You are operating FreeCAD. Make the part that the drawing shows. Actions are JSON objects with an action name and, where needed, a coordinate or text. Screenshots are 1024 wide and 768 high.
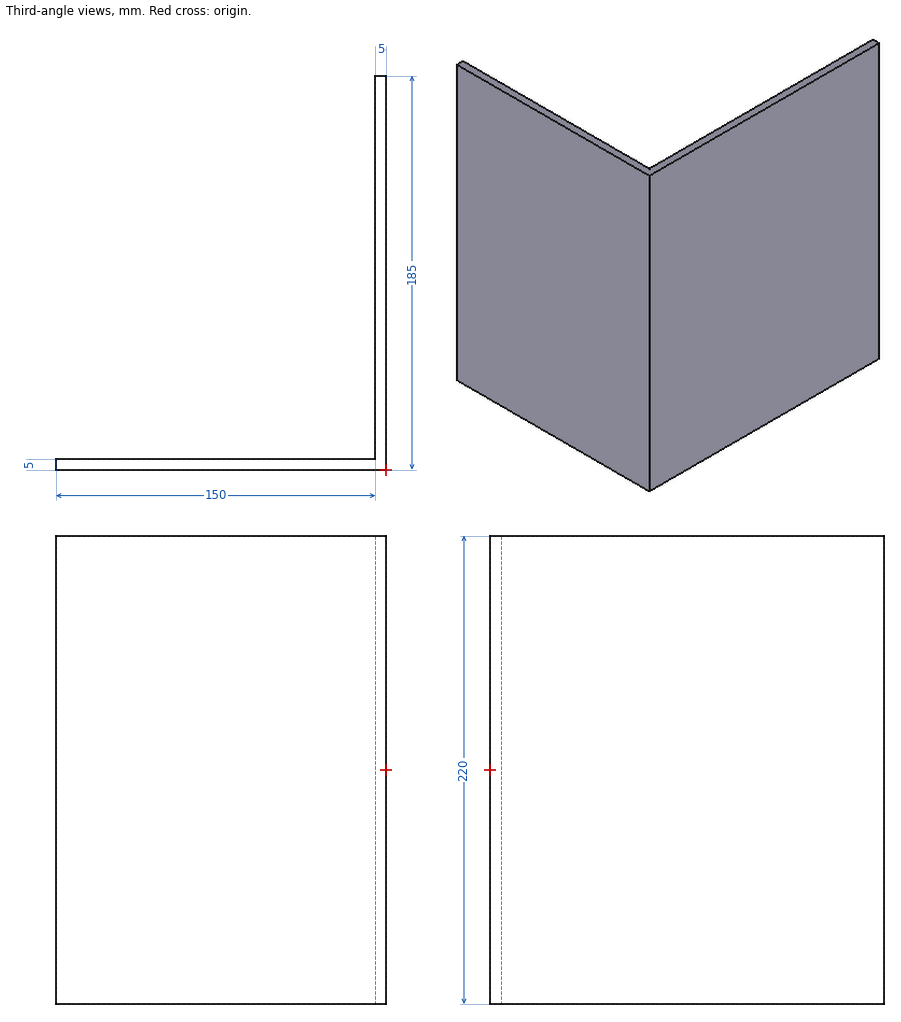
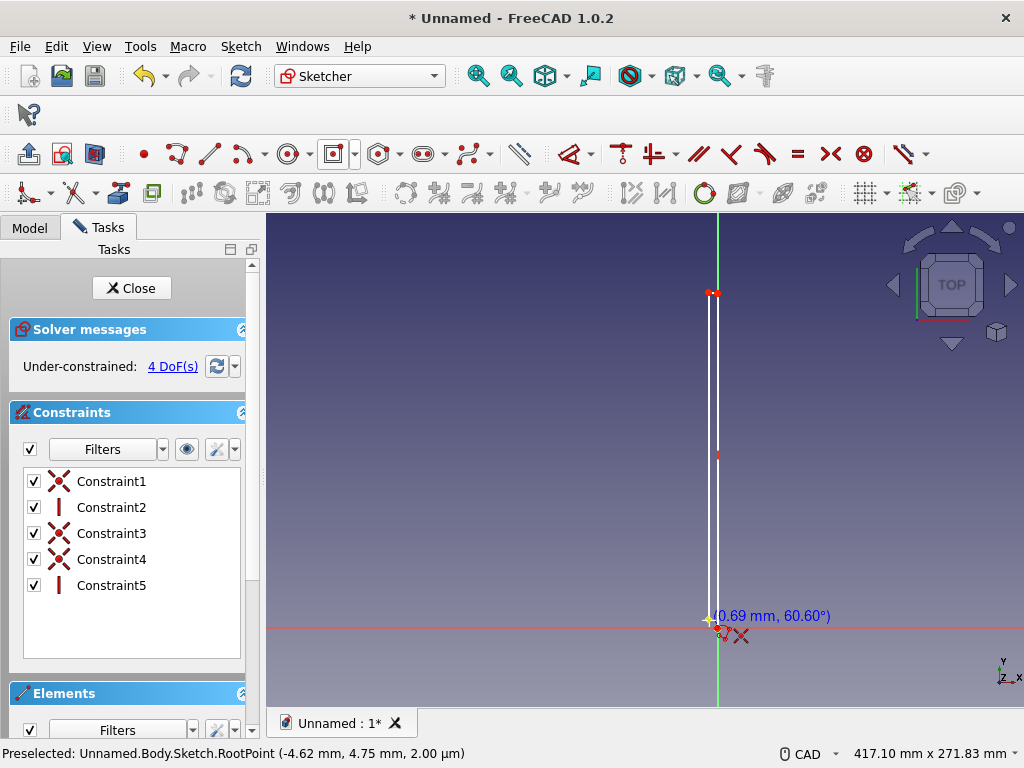
{"action": "scroll", "coordinate": [436, 619], "scroll_direction": "up", "scroll_amount": 3}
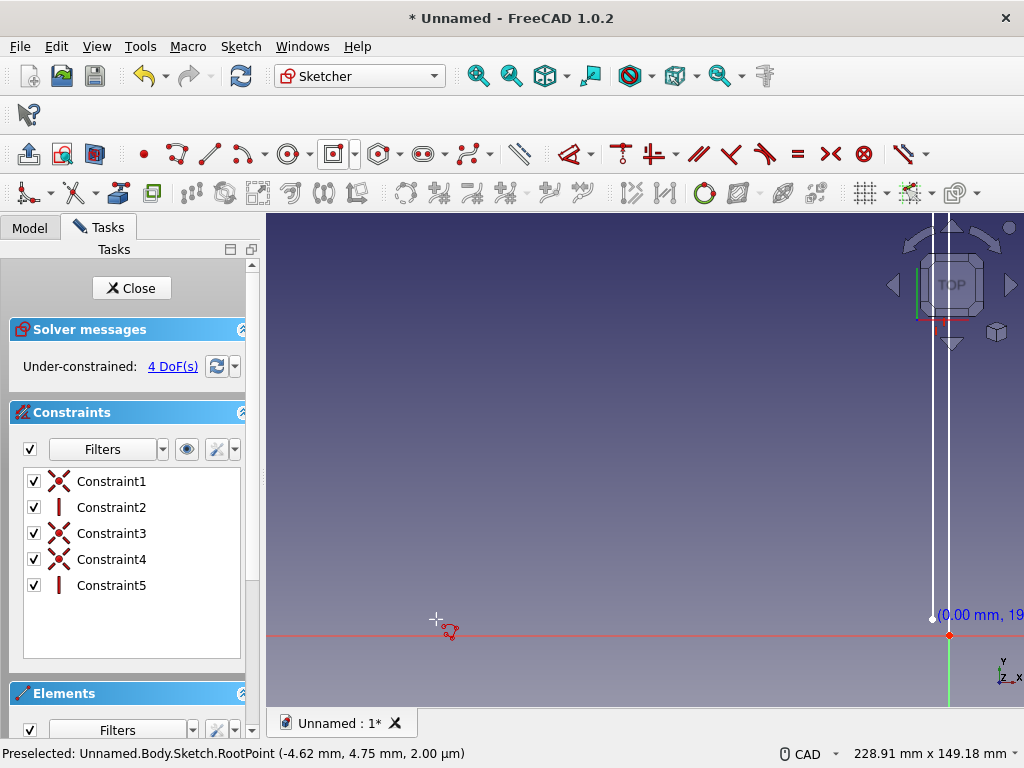
{"action": "left_click", "coordinate": [436, 619]}
{"action": "left_click", "coordinate": [436, 627]}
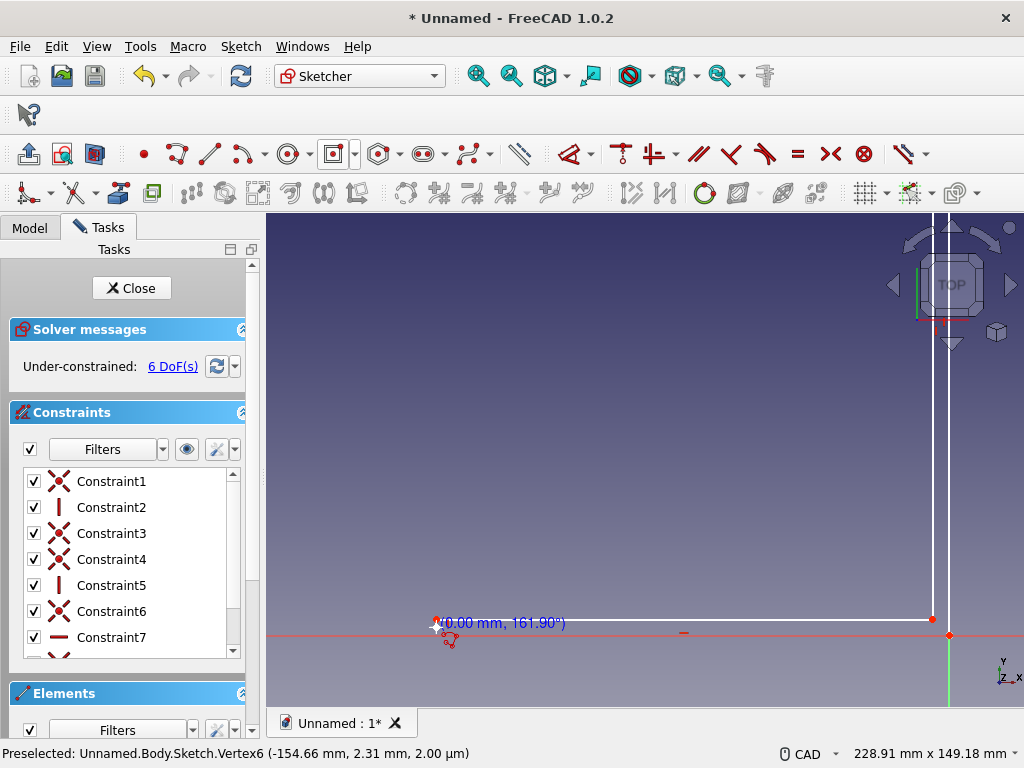
{"action": "scroll", "coordinate": [436, 619], "scroll_direction": "down", "scroll_amount": 3}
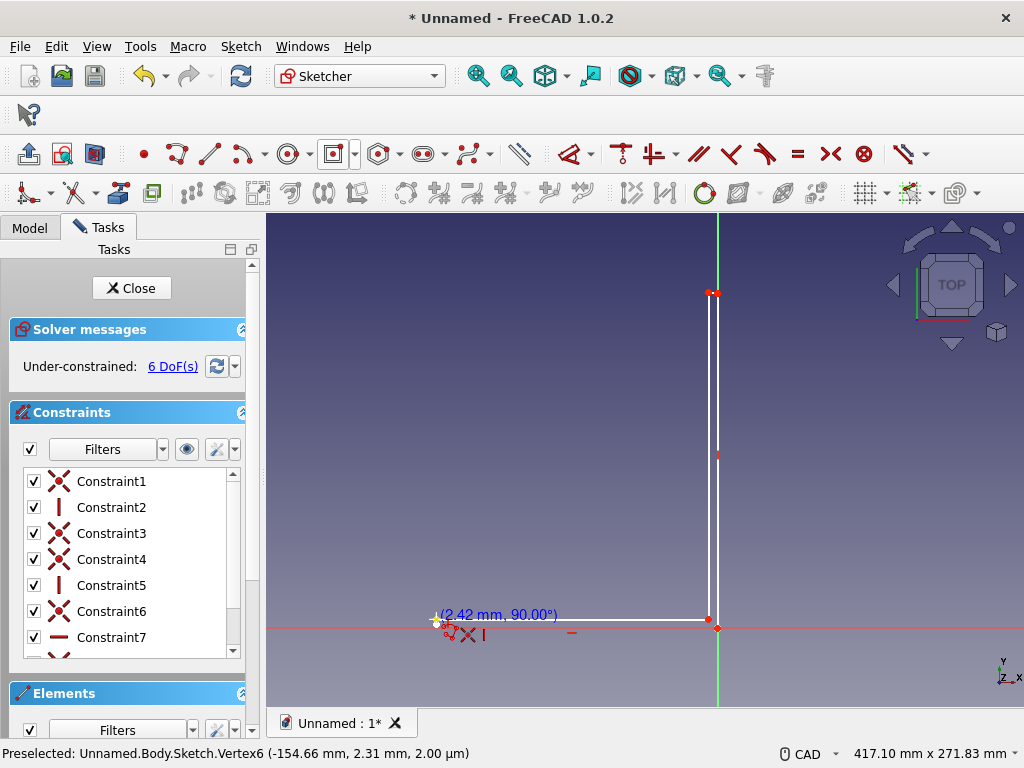
{"action": "scroll", "coordinate": [718, 628], "scroll_direction": "up", "scroll_amount": 2}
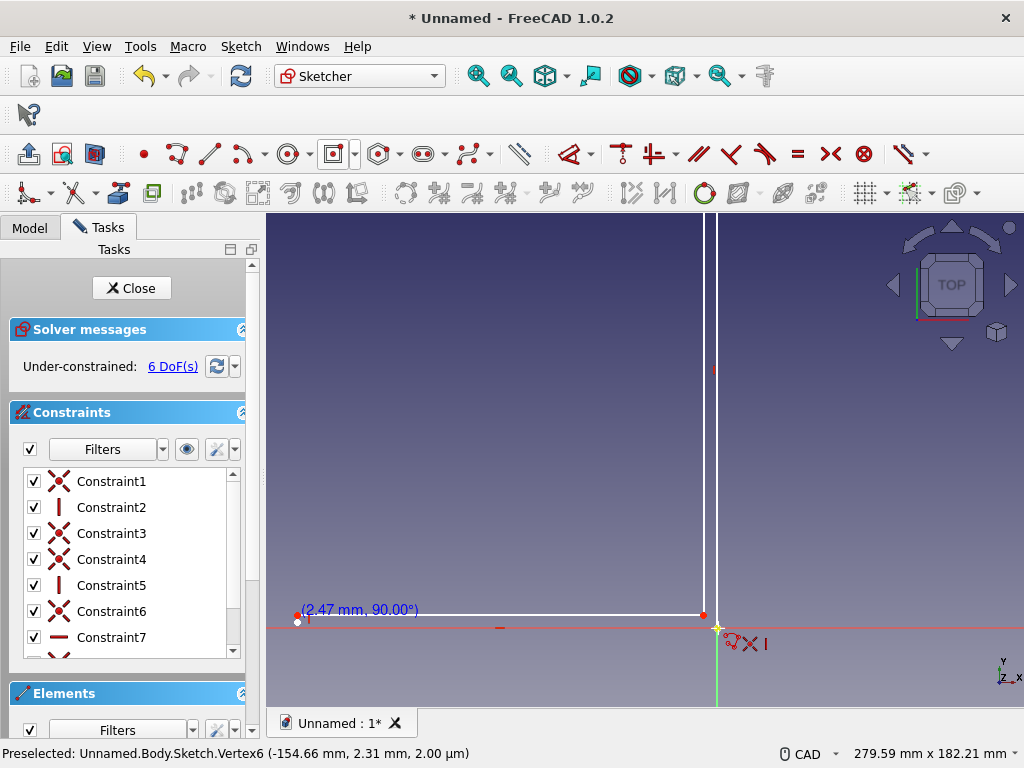
{"action": "left_click", "coordinate": [717, 628]}
{"action": "key", "text": "Escape"}
{"action": "key", "text": "Escape"}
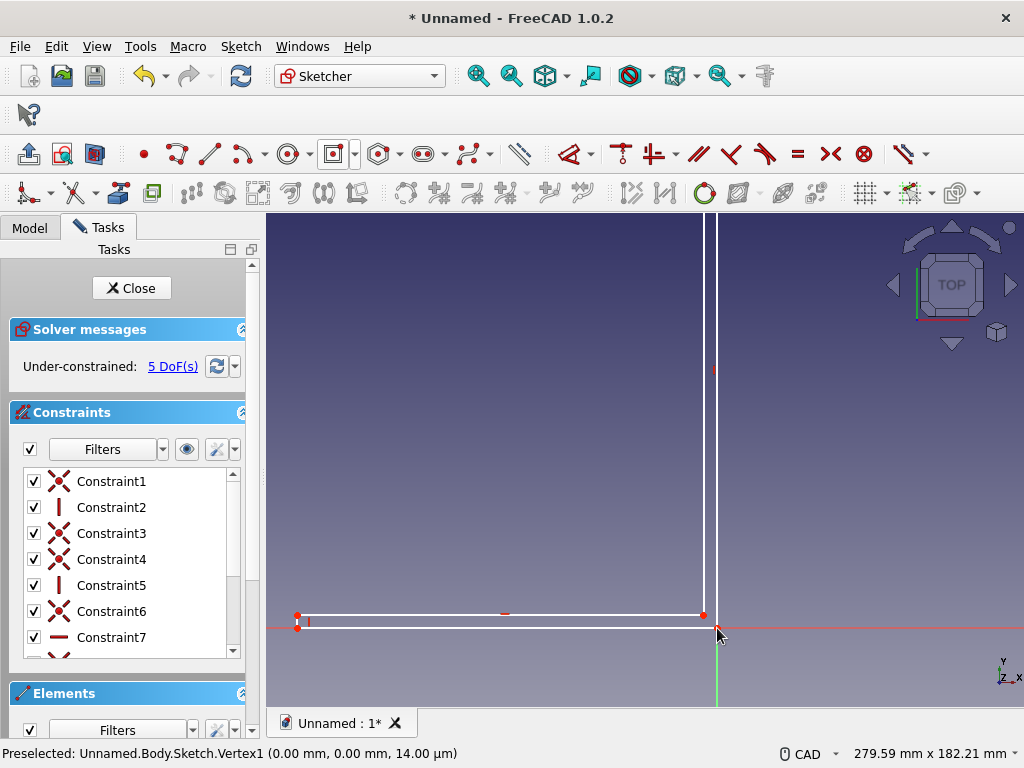
{"action": "scroll", "coordinate": [718, 628], "scroll_direction": "down", "scroll_amount": 2}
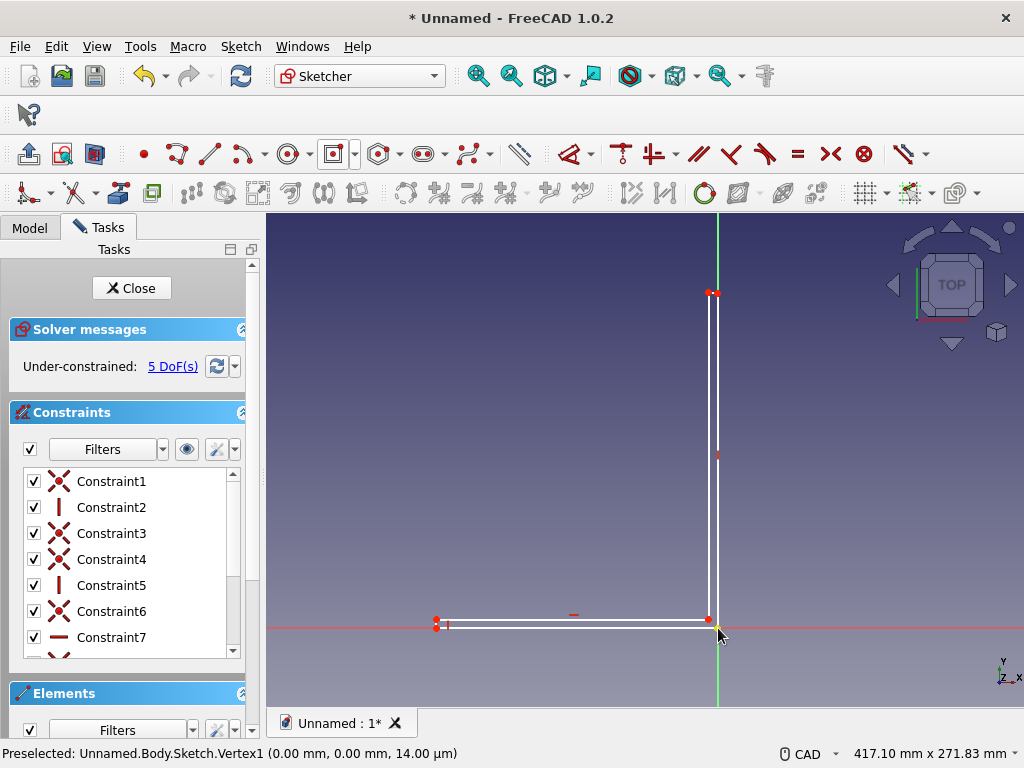
{"action": "scroll", "coordinate": [713, 293], "scroll_direction": "up", "scroll_amount": 6}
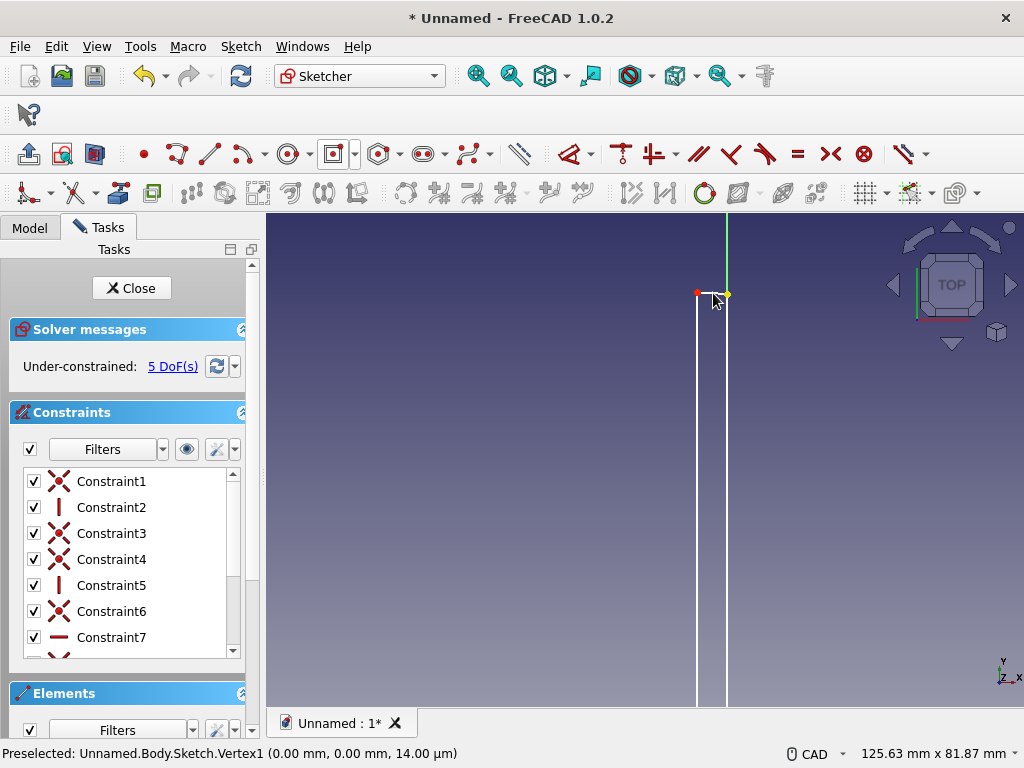
{"action": "left_click", "coordinate": [712, 293]}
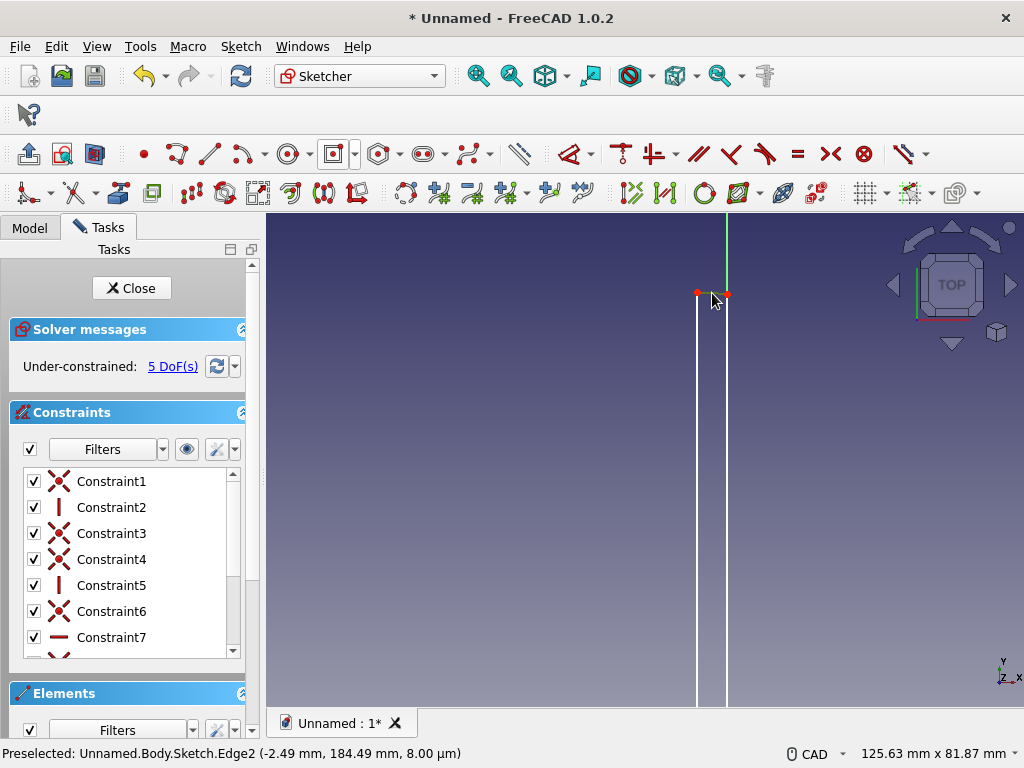
{"action": "left_click", "coordinate": [676, 154]}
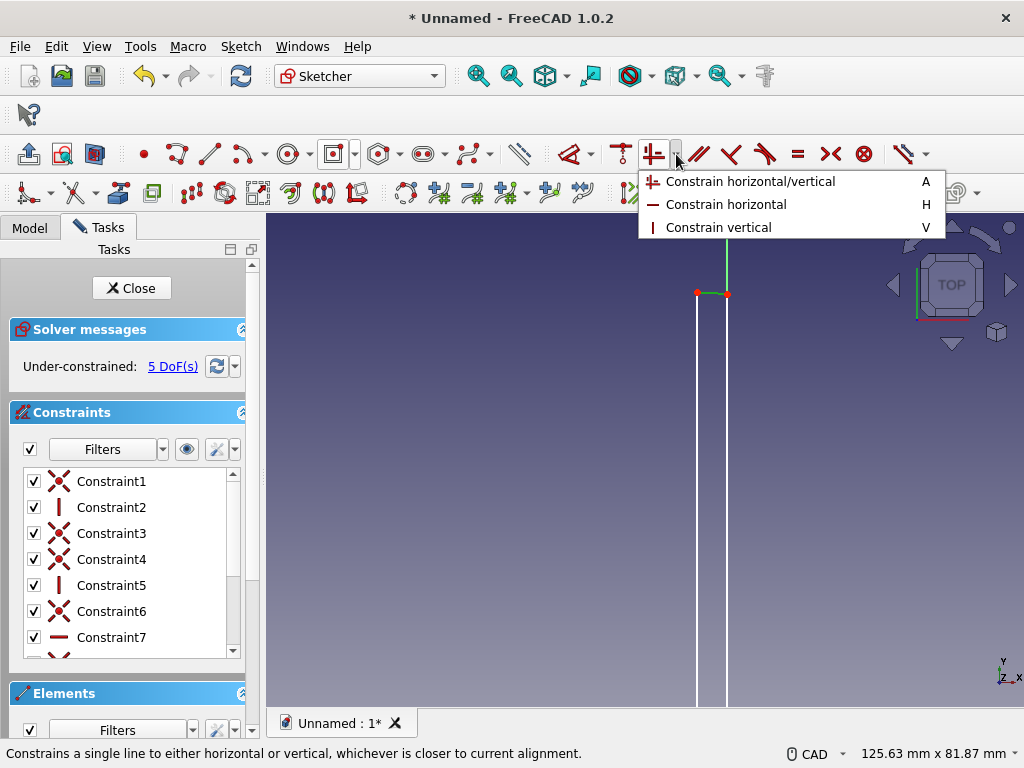
{"action": "left_click", "coordinate": [792, 204]}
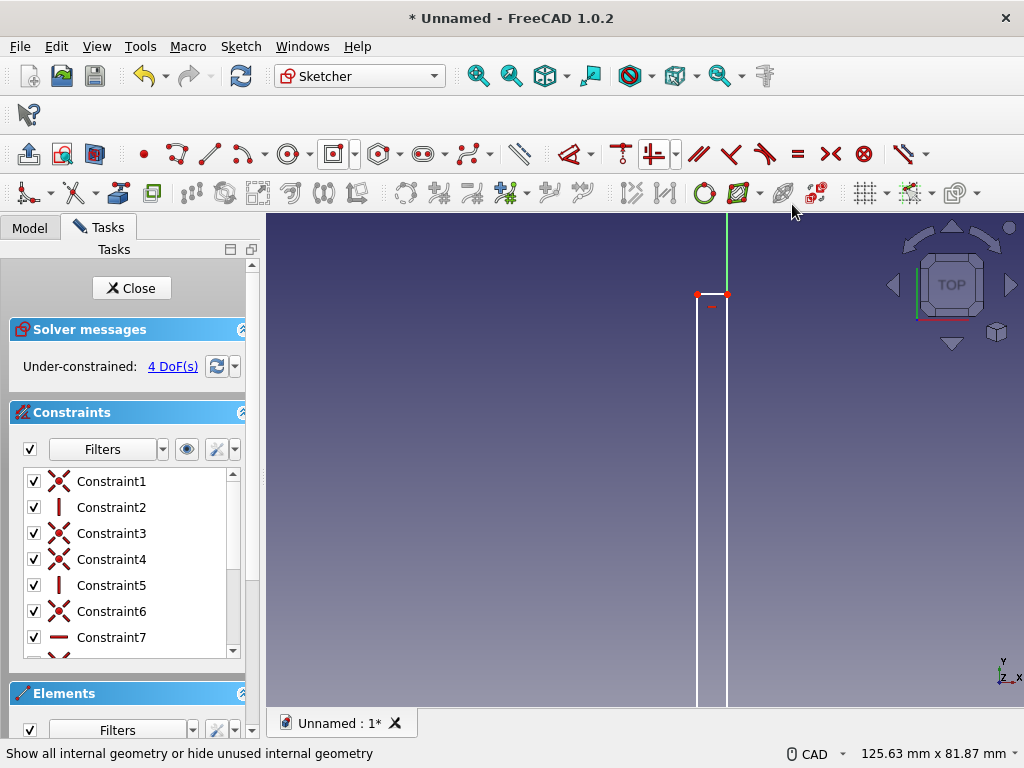
{"action": "left_click", "coordinate": [568, 154]}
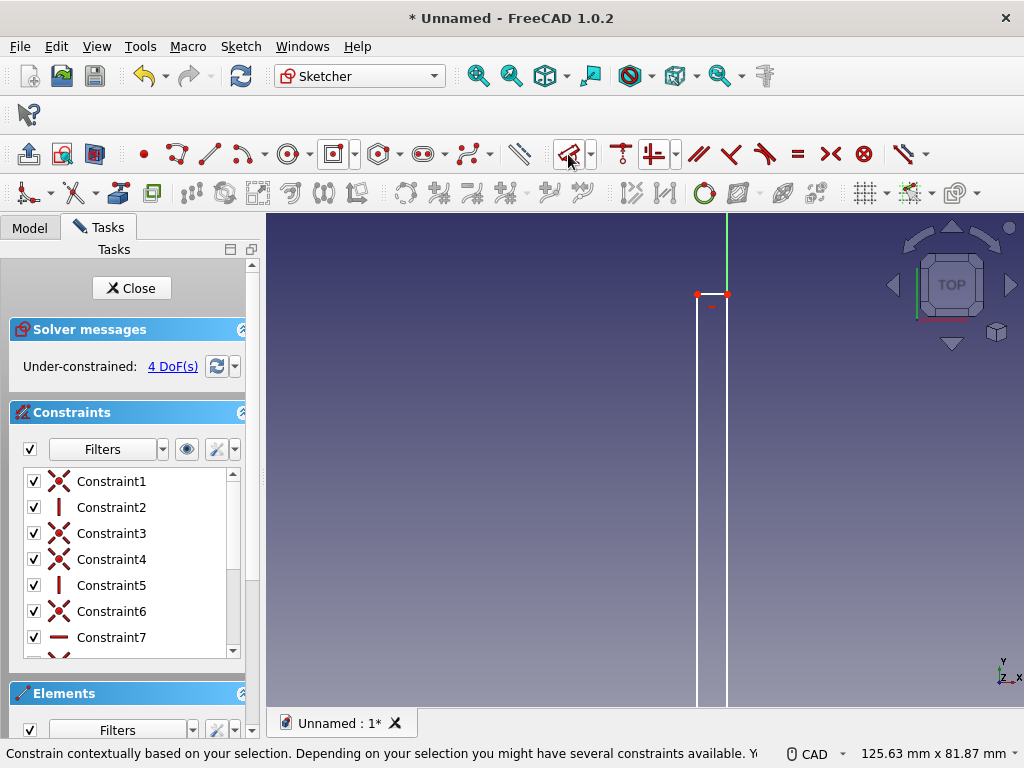
{"action": "scroll", "coordinate": [715, 294], "scroll_direction": "up", "scroll_amount": 2}